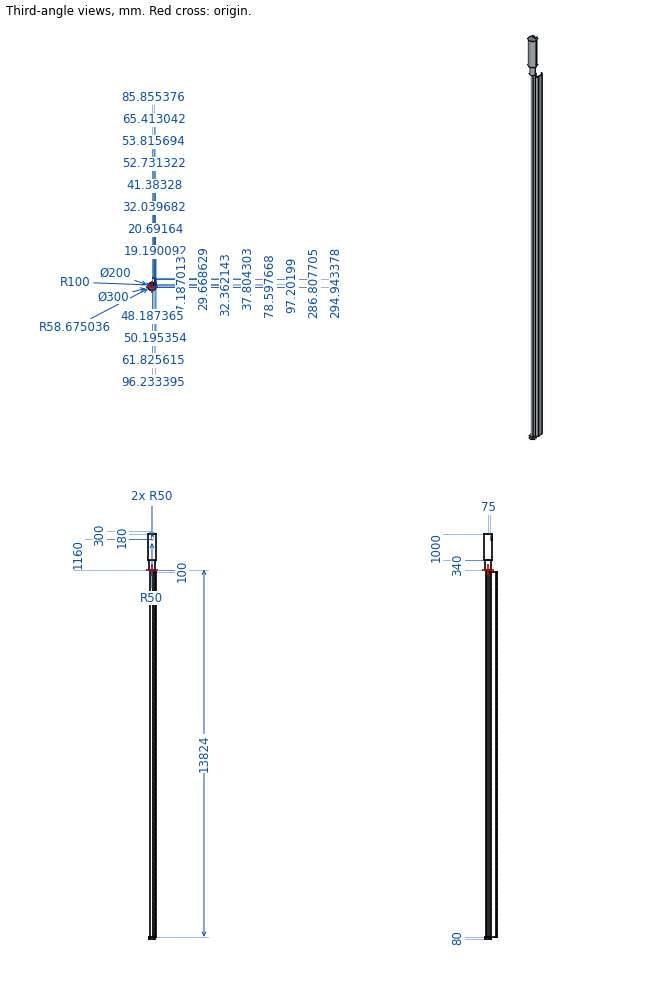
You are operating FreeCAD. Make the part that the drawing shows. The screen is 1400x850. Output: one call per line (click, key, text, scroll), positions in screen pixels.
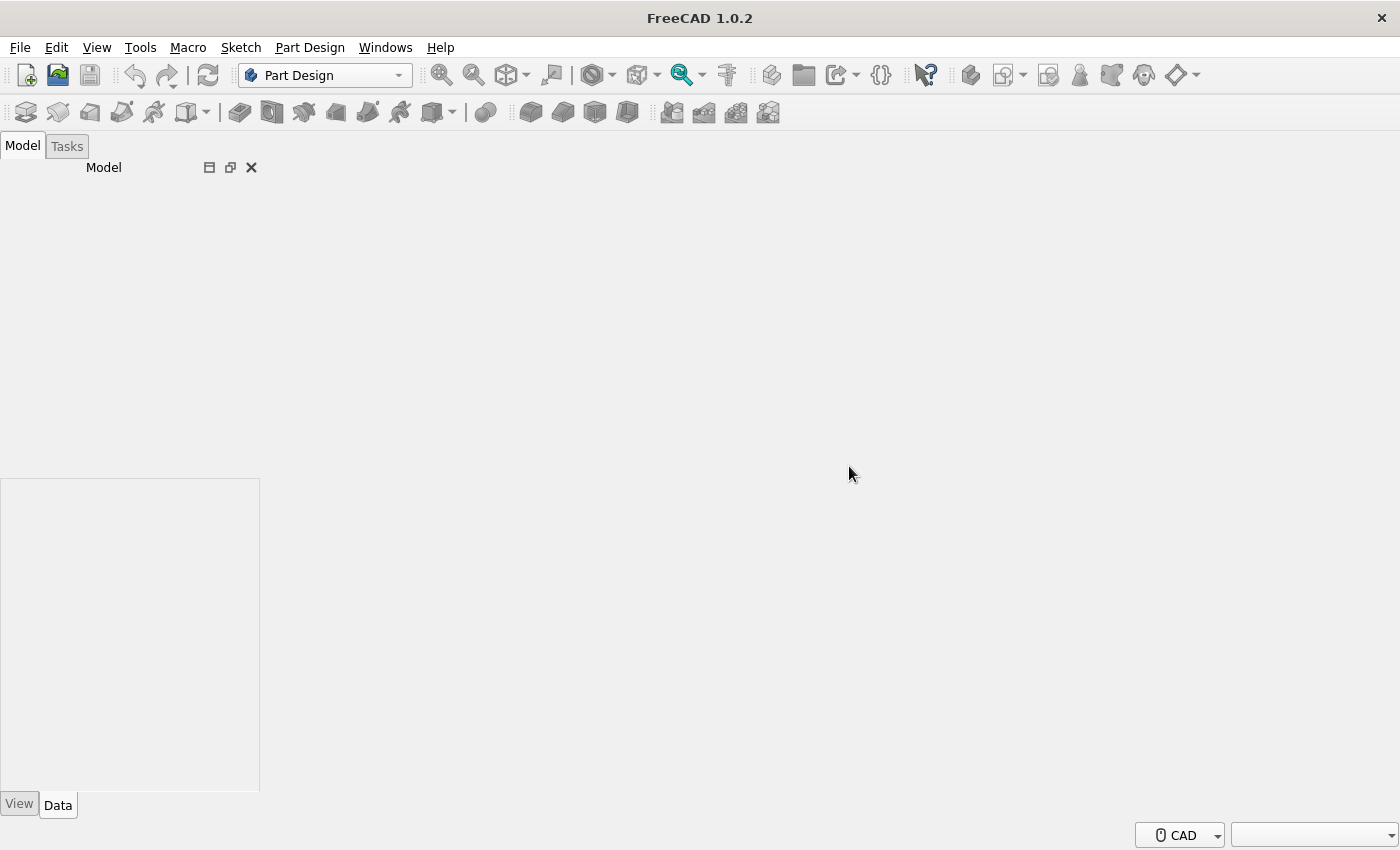
key(ctrl+n)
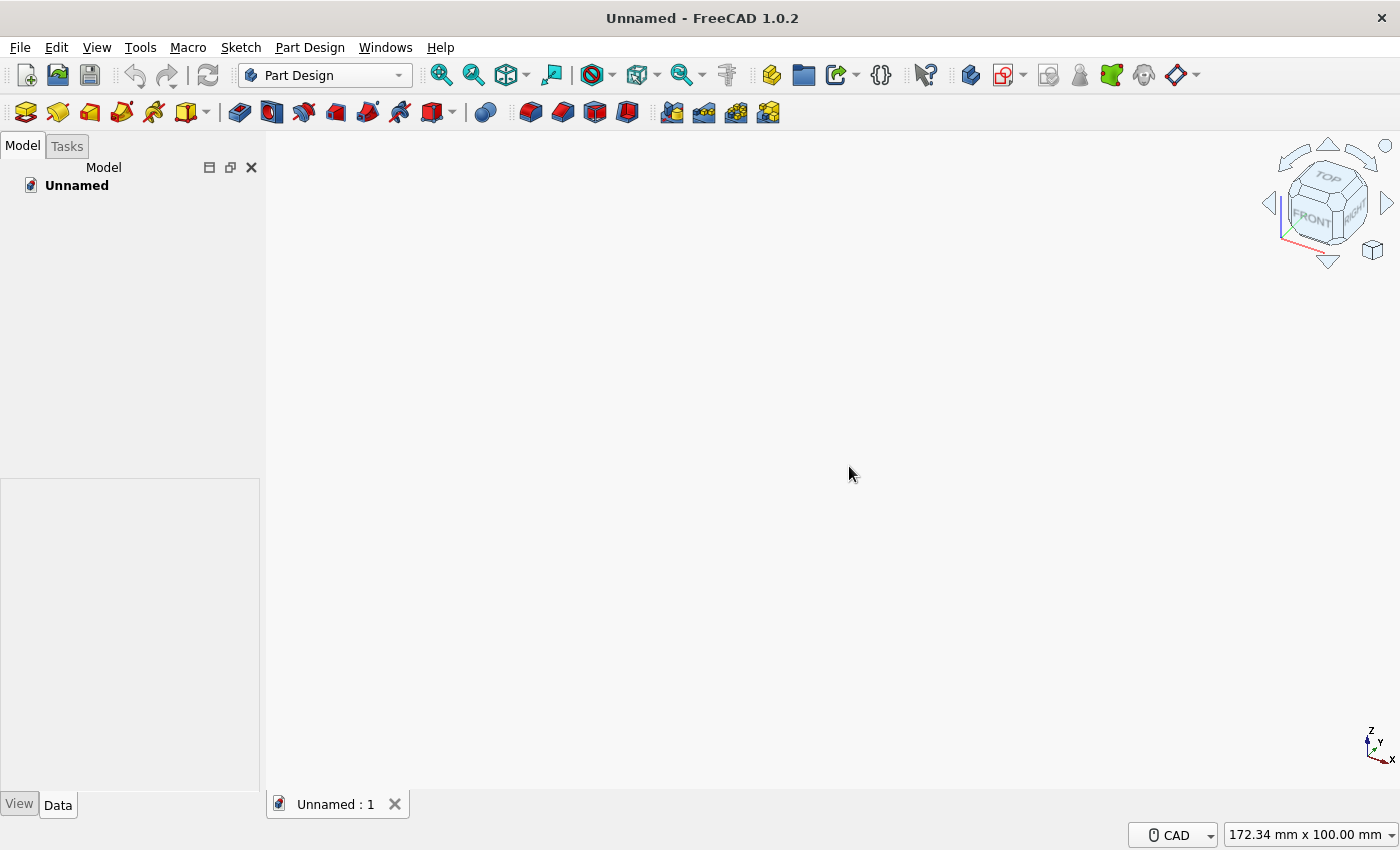
click(1004, 76)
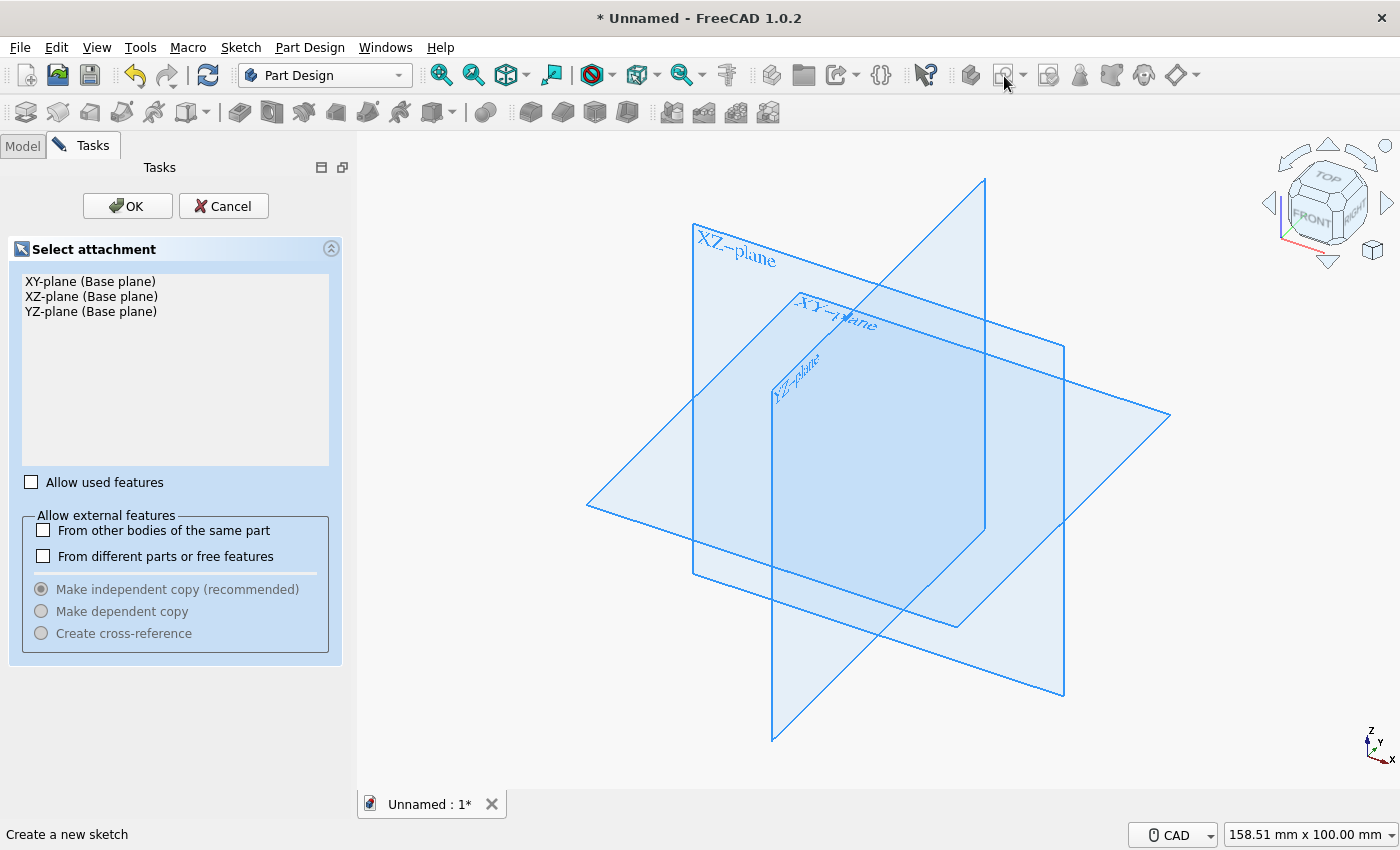
click(82, 282)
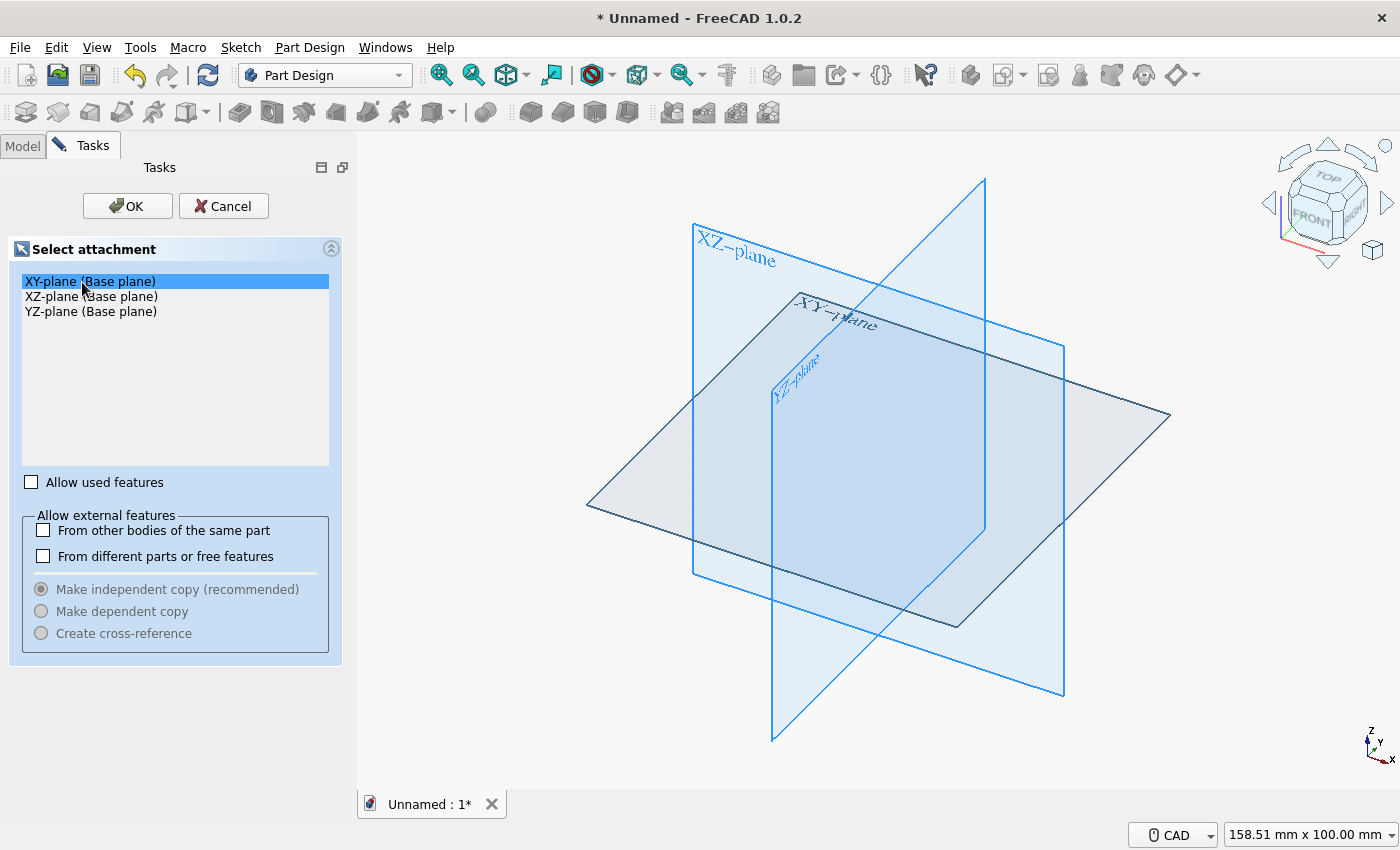
click(128, 206)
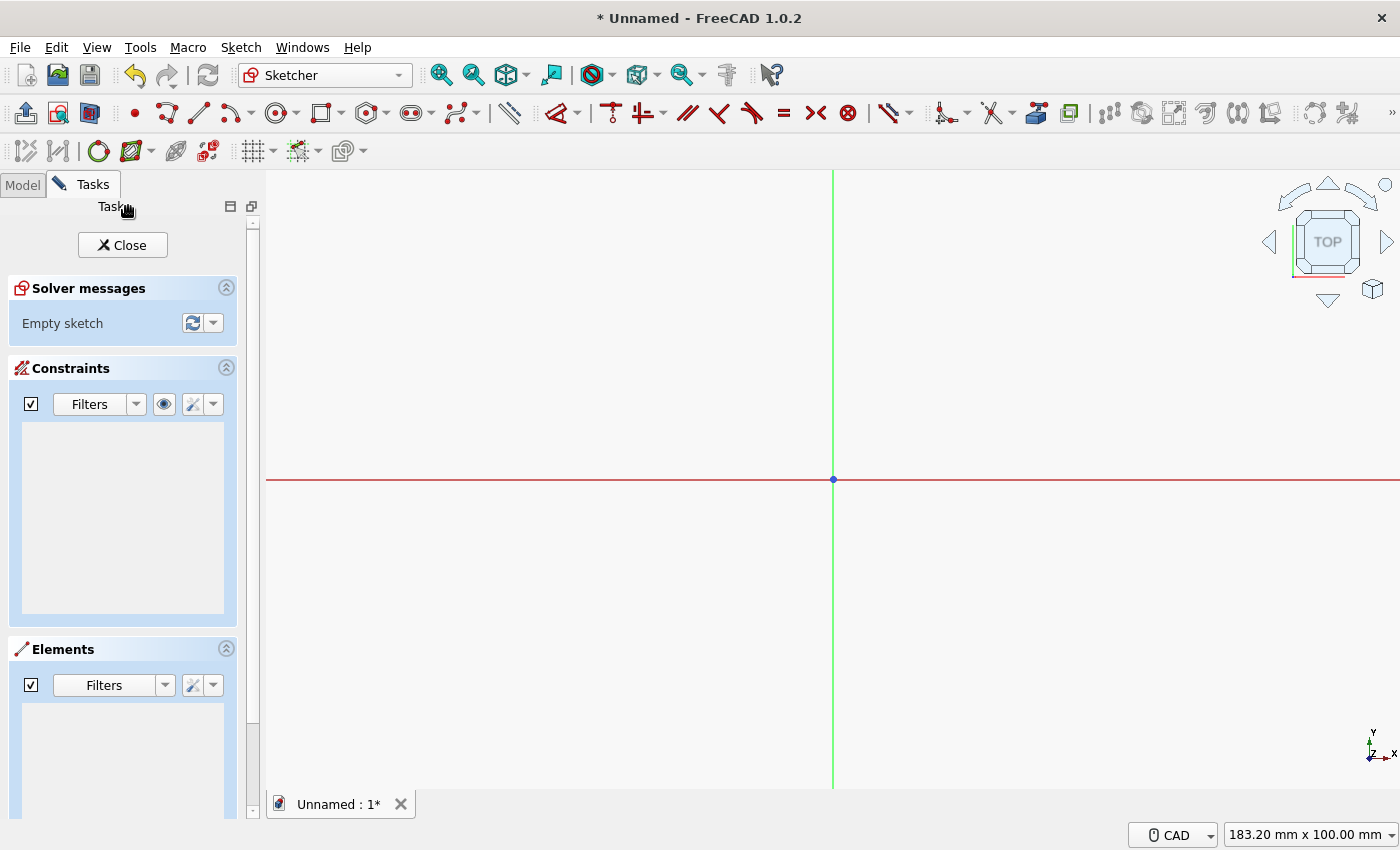
scroll(735, 480, down, 6)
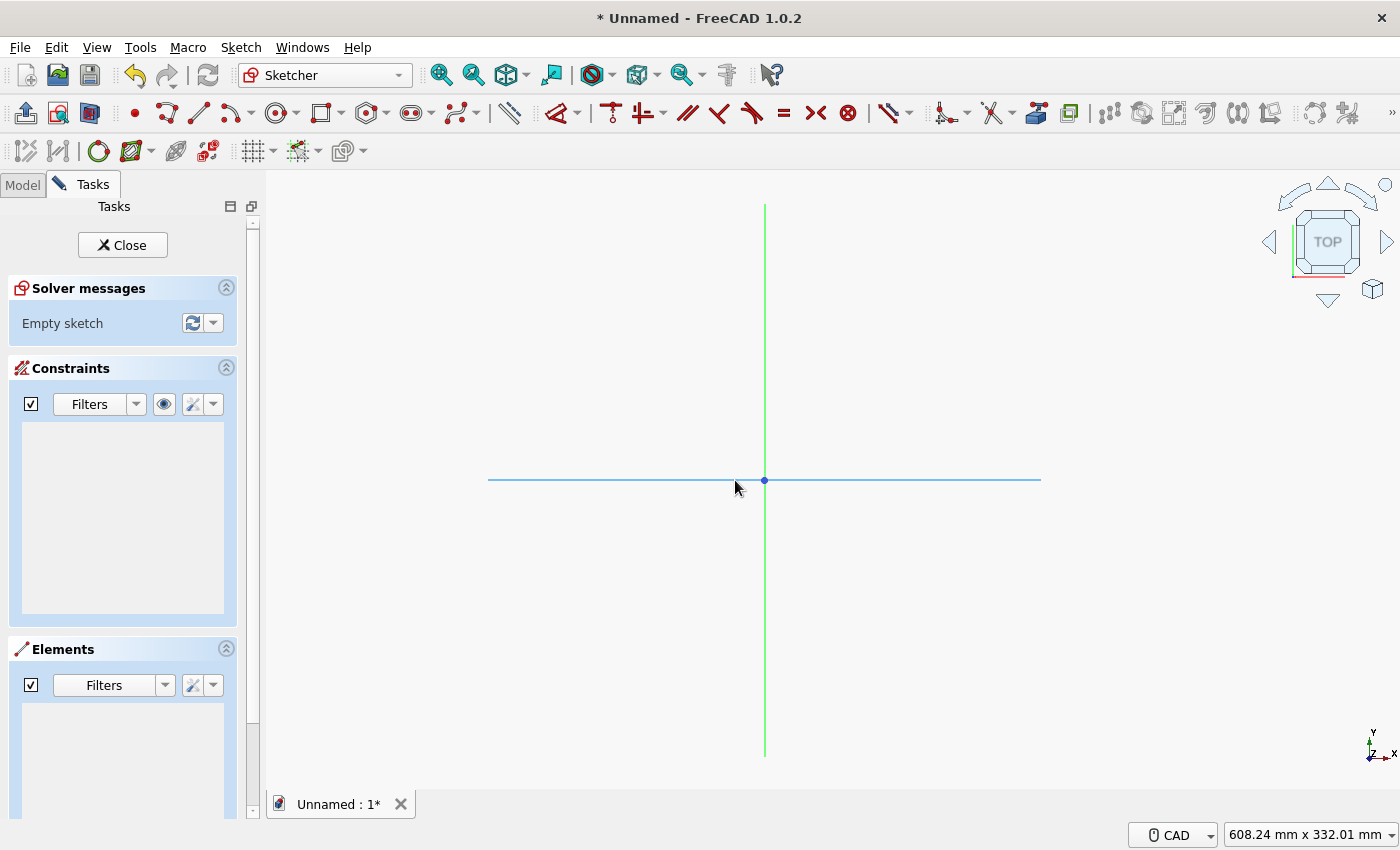
key(g)
key(c)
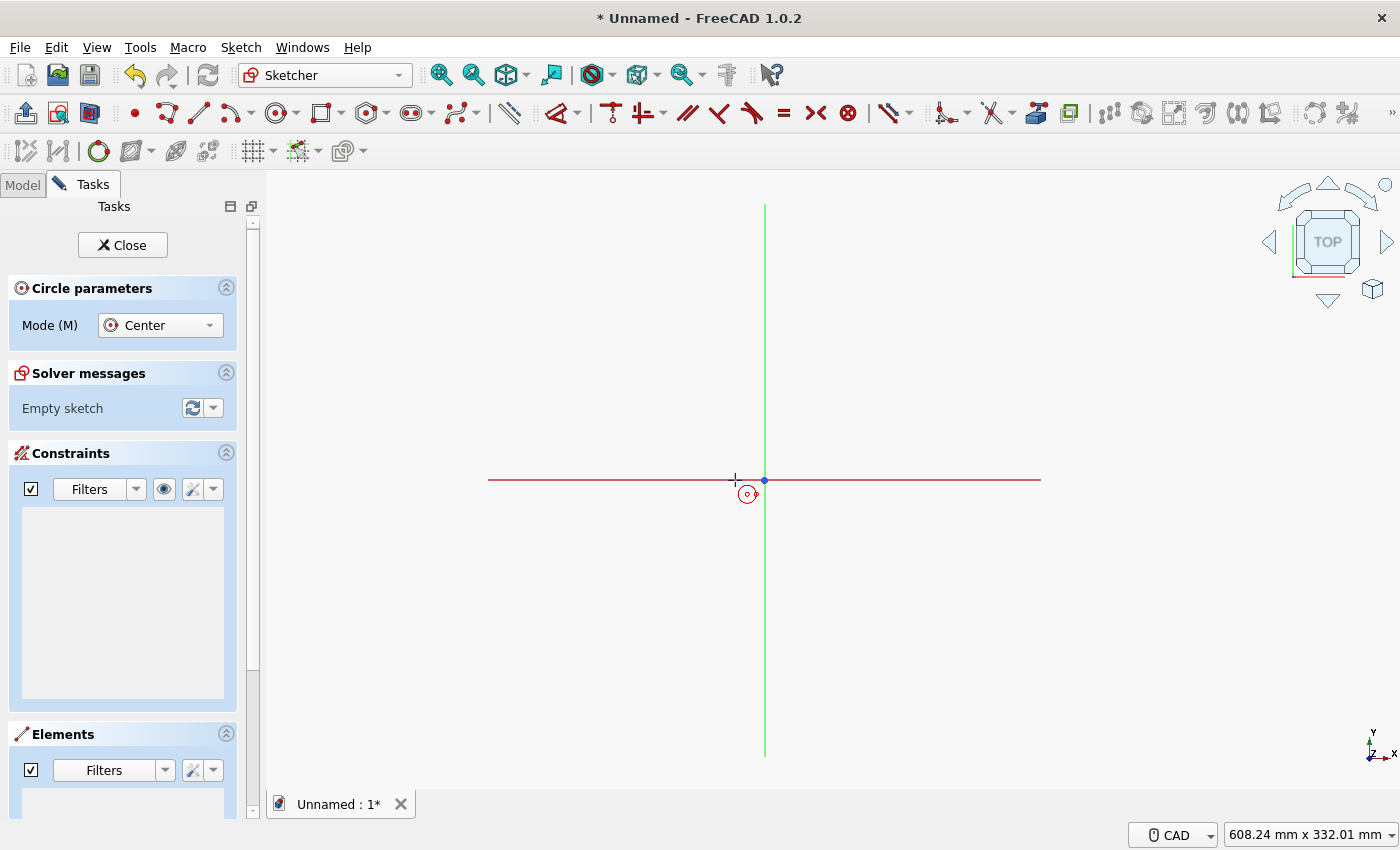
click(765, 480)
click(897, 348)
key(Escape)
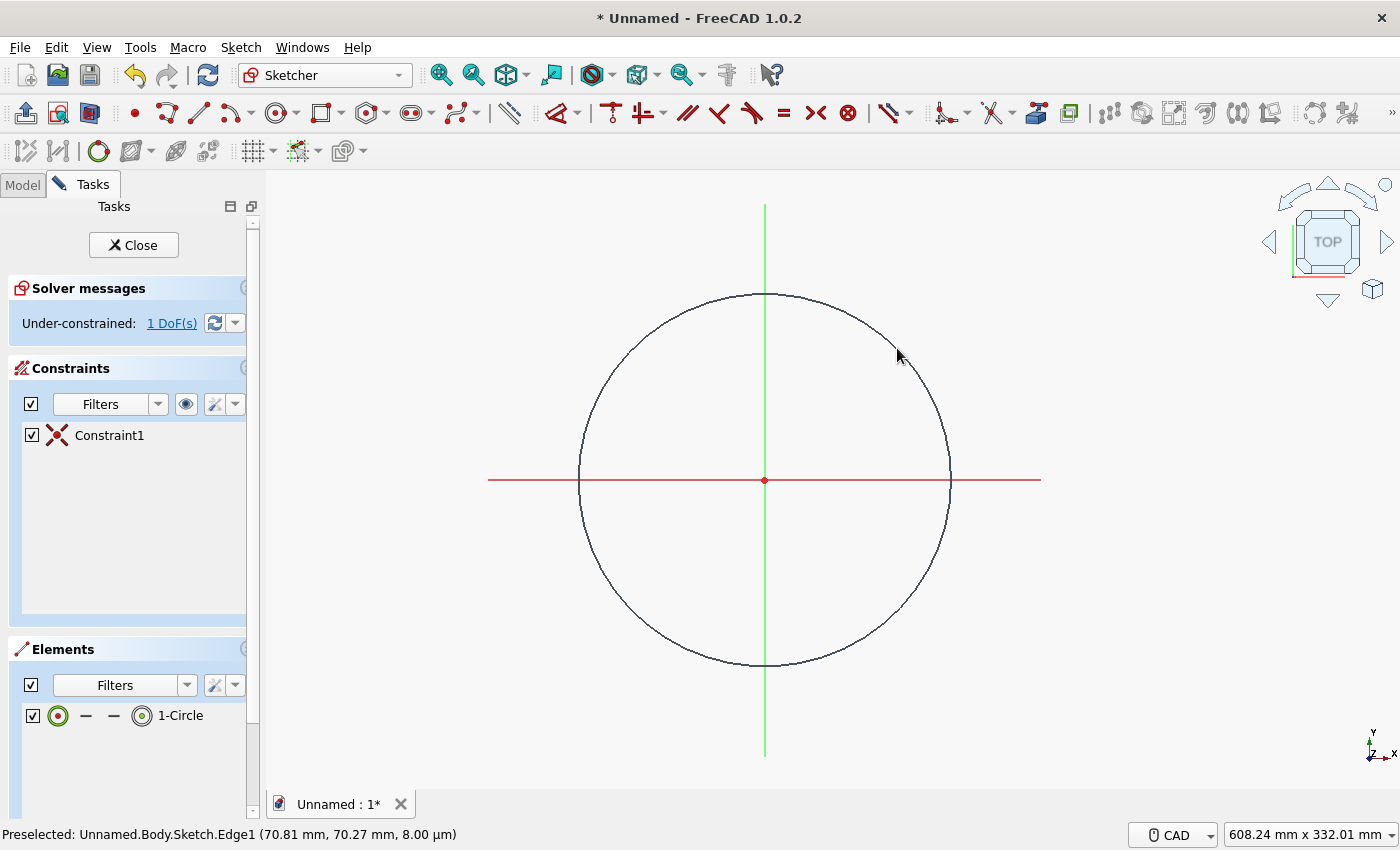
key(d)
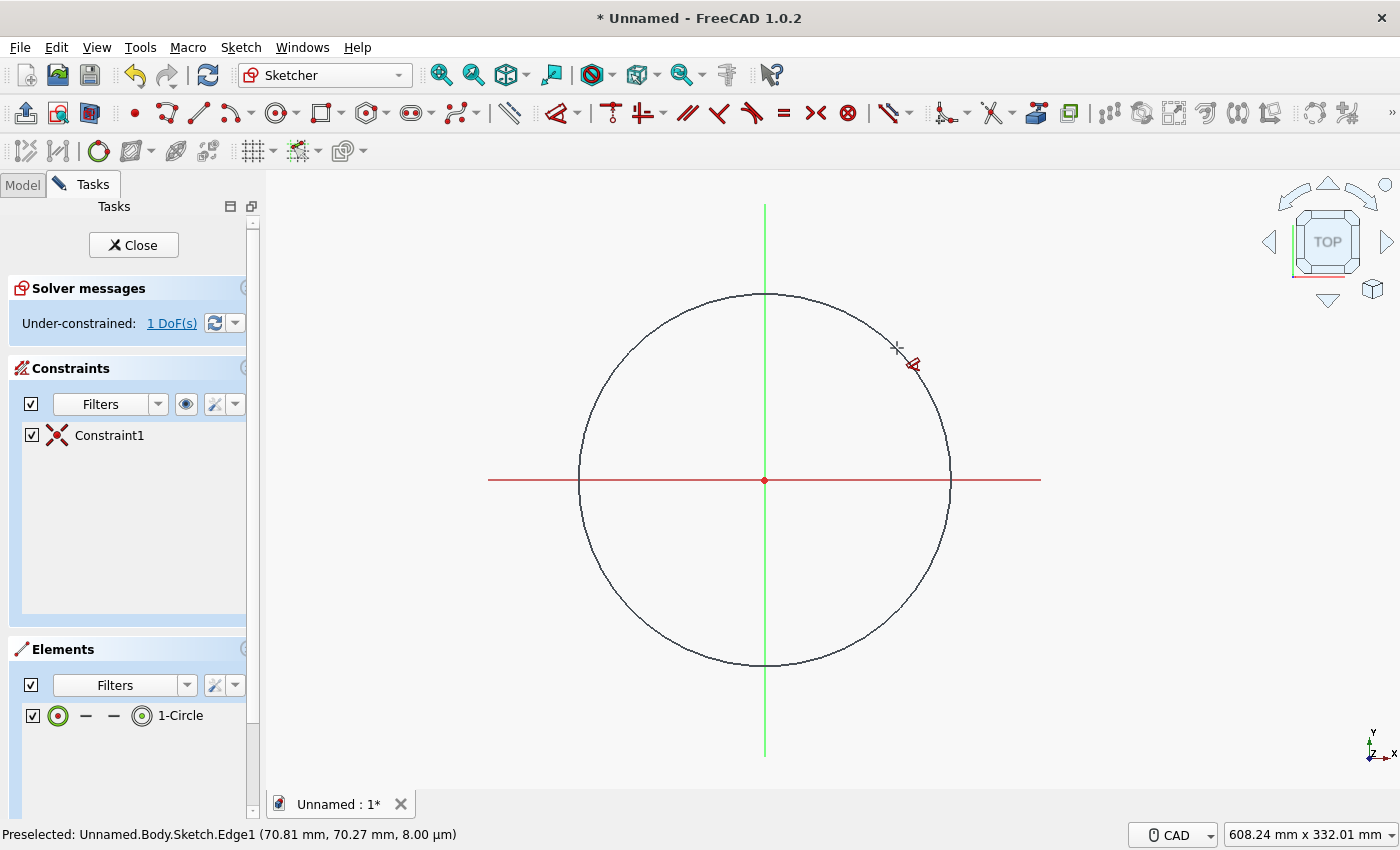
click(896, 348)
click(919, 325)